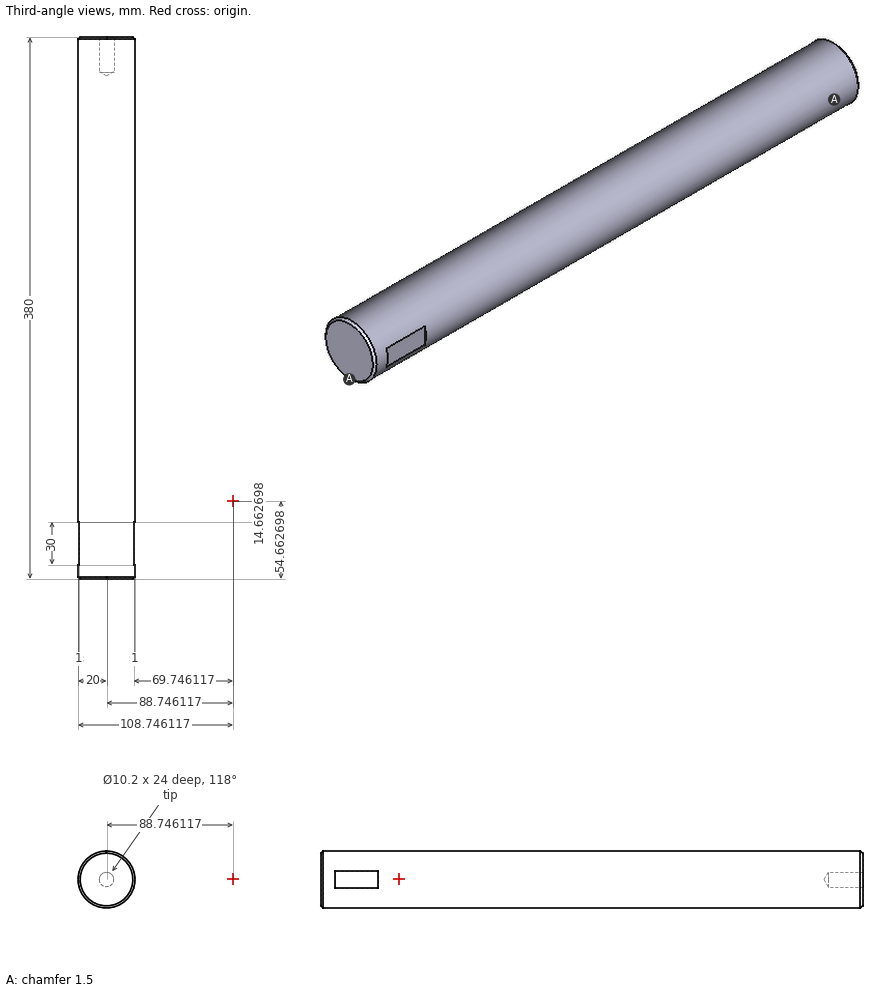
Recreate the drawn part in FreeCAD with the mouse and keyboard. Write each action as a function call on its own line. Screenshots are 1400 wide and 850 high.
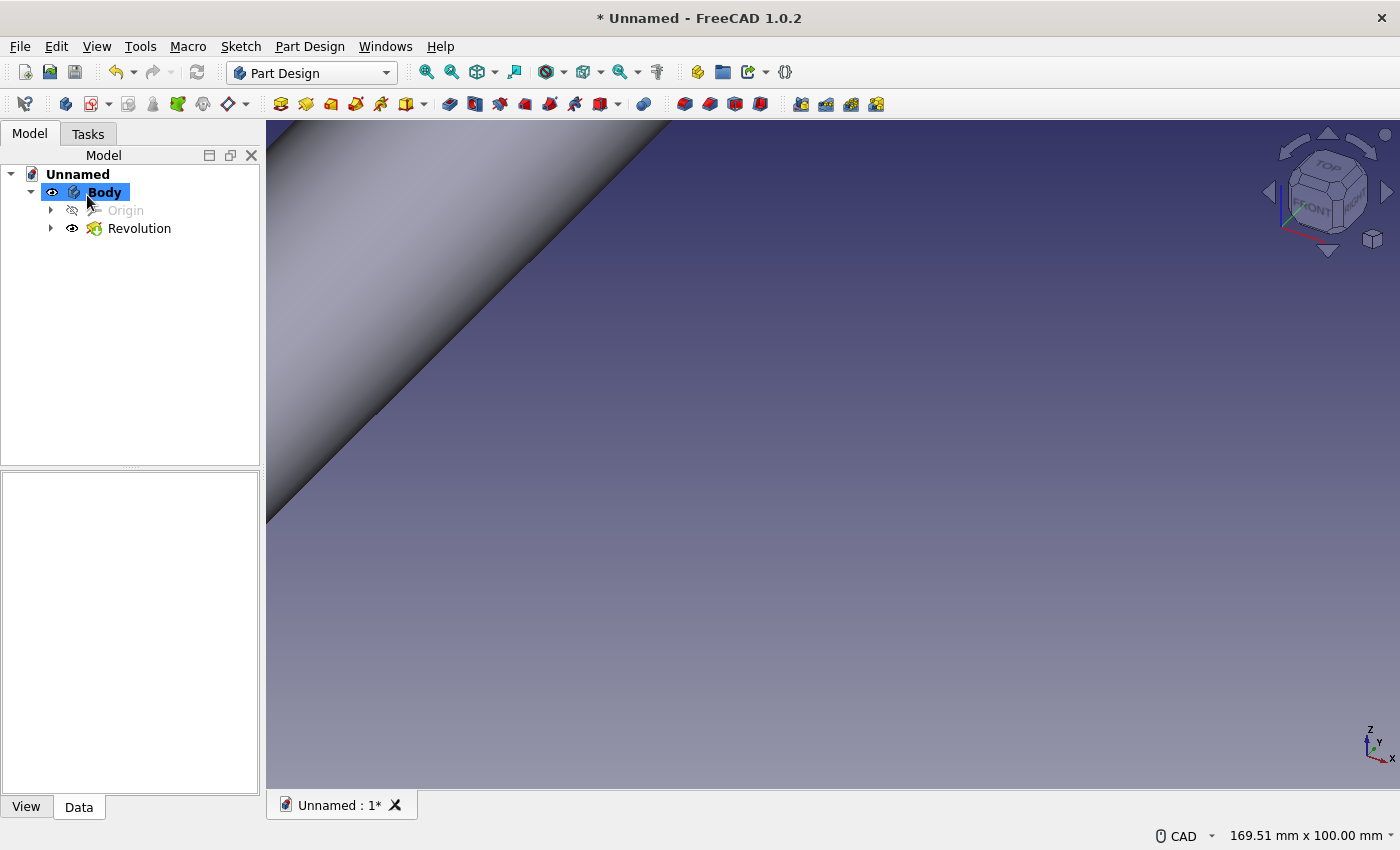
click(427, 72)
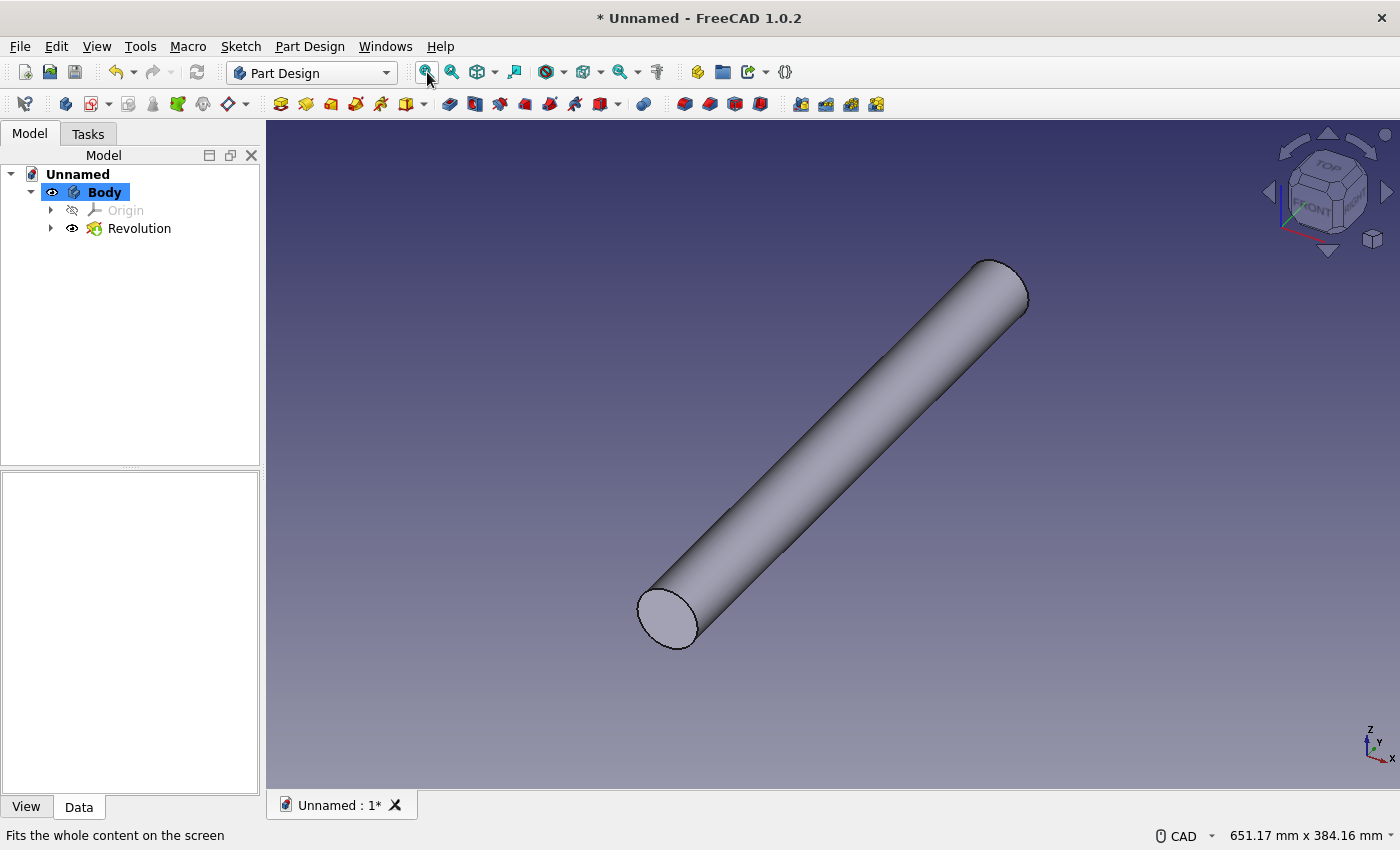
click(90, 104)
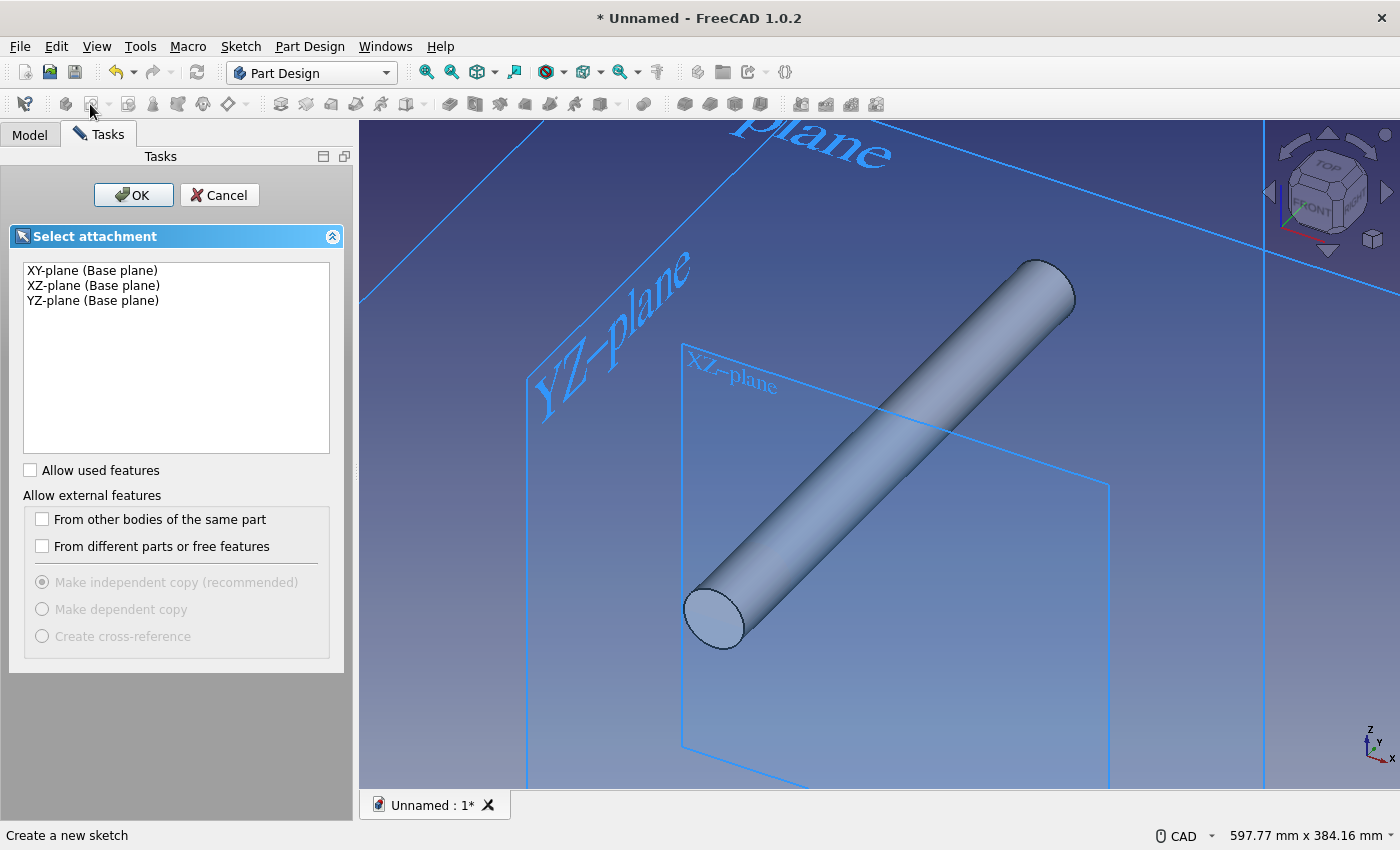
click(84, 270)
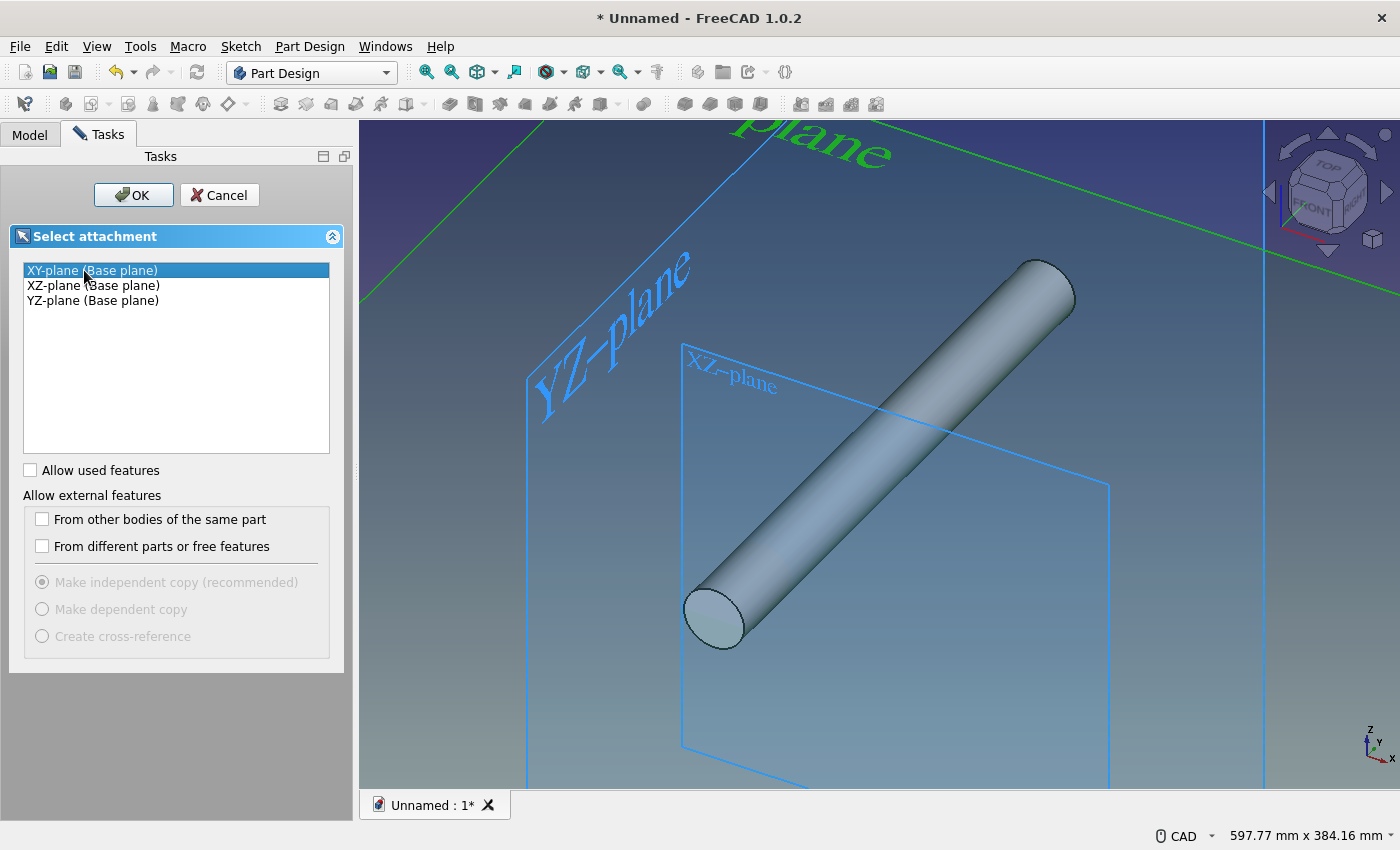
click(134, 195)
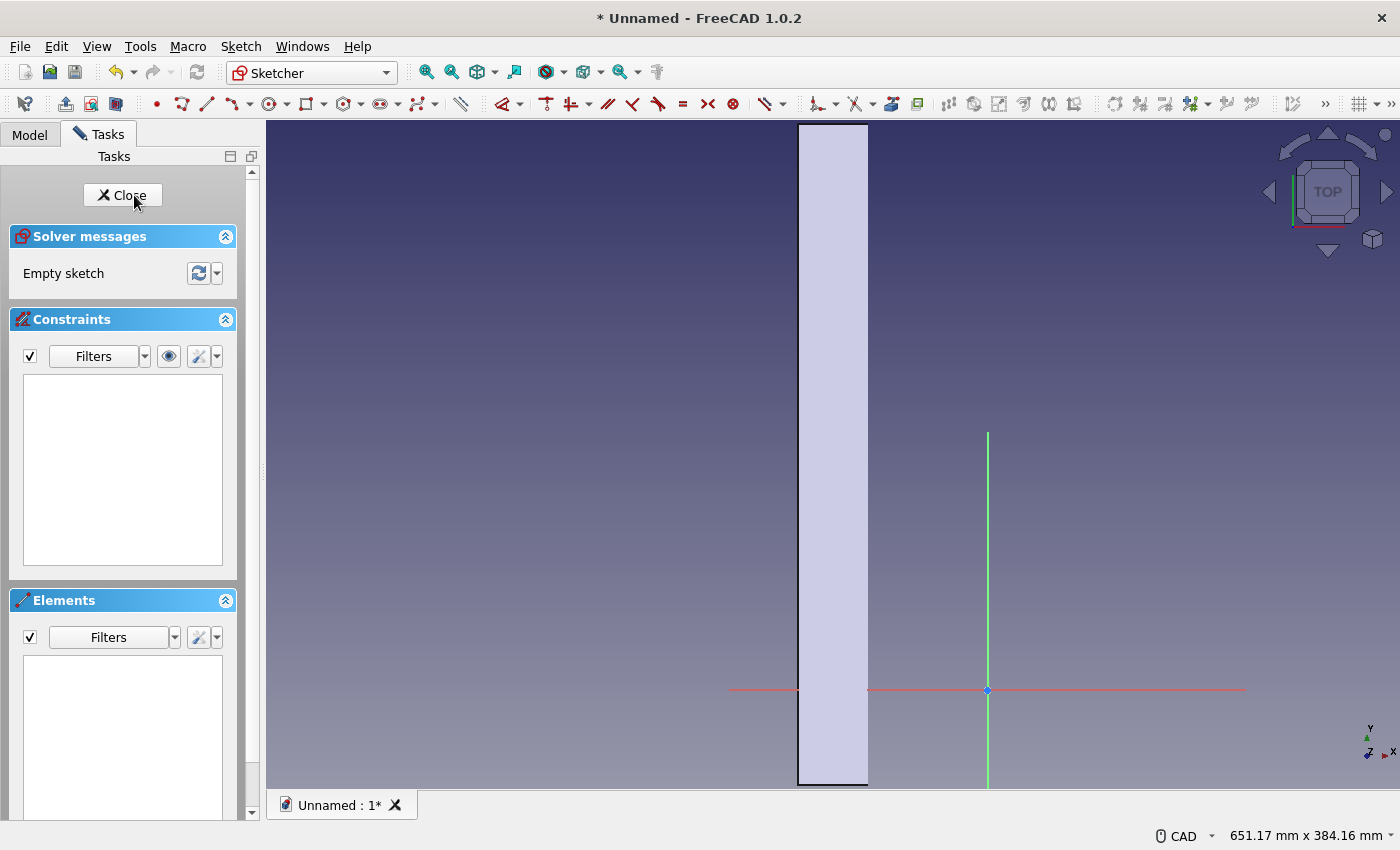
click(116, 104)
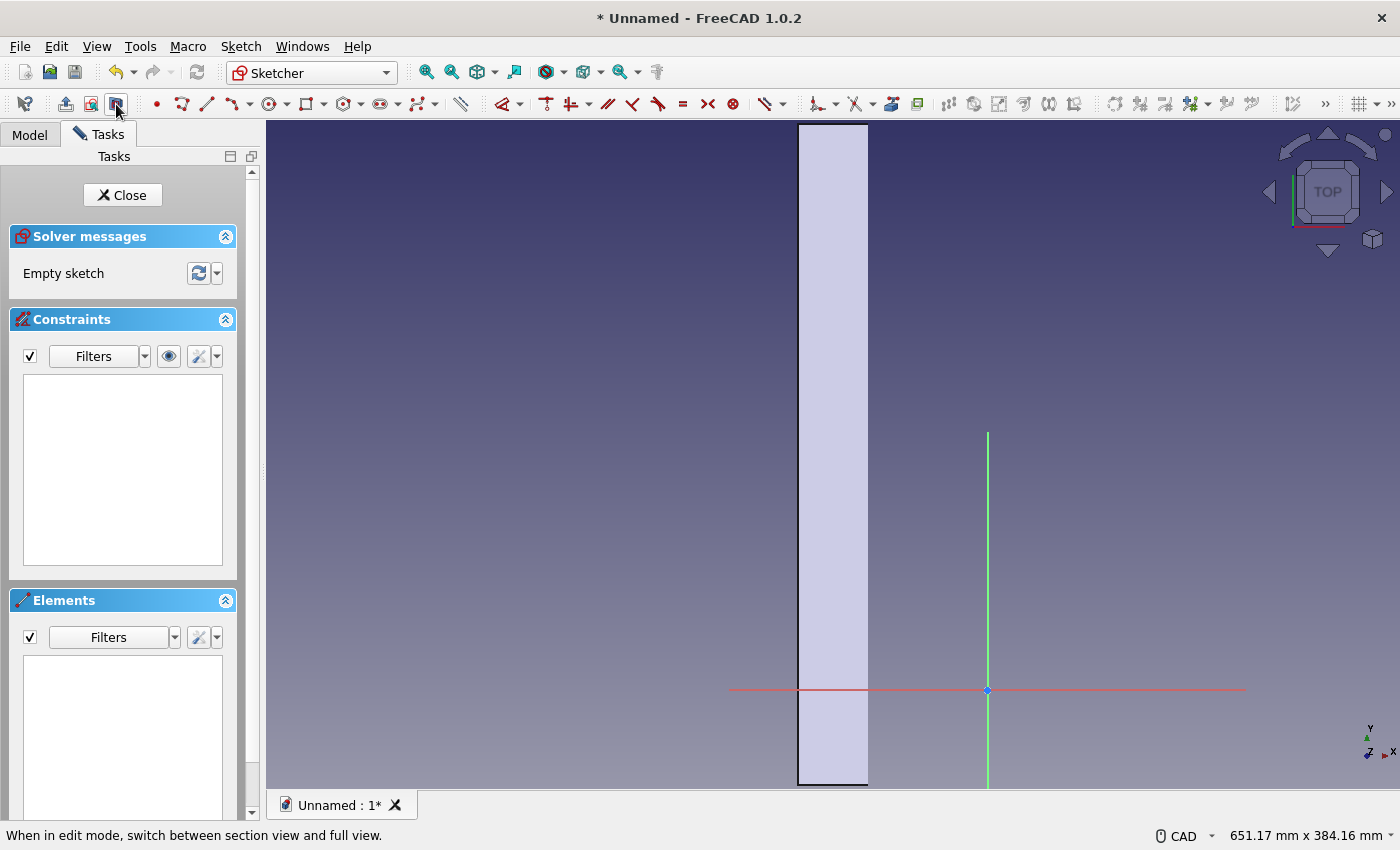
scroll(764, 454, down, 5)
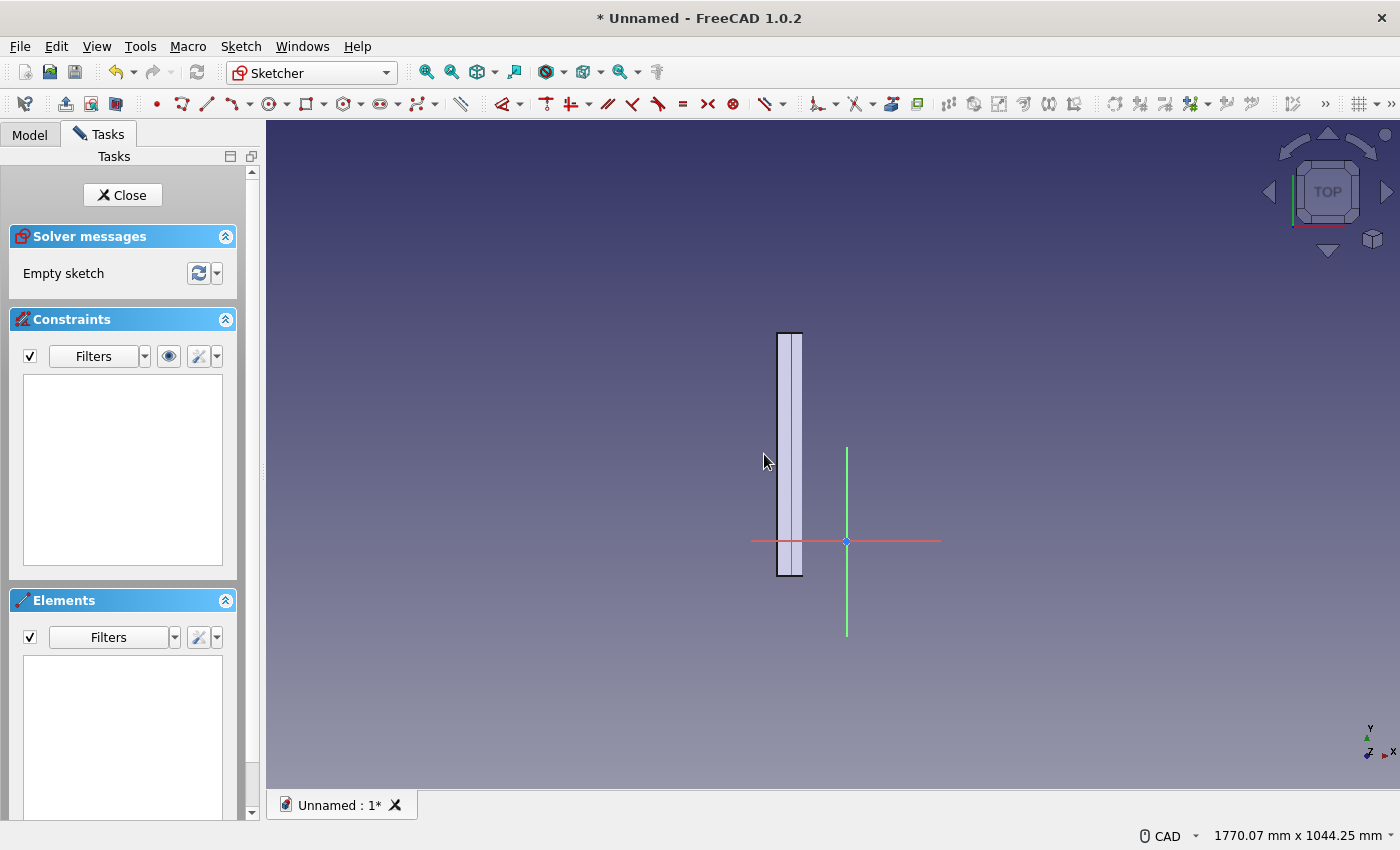
scroll(791, 566, up, 15)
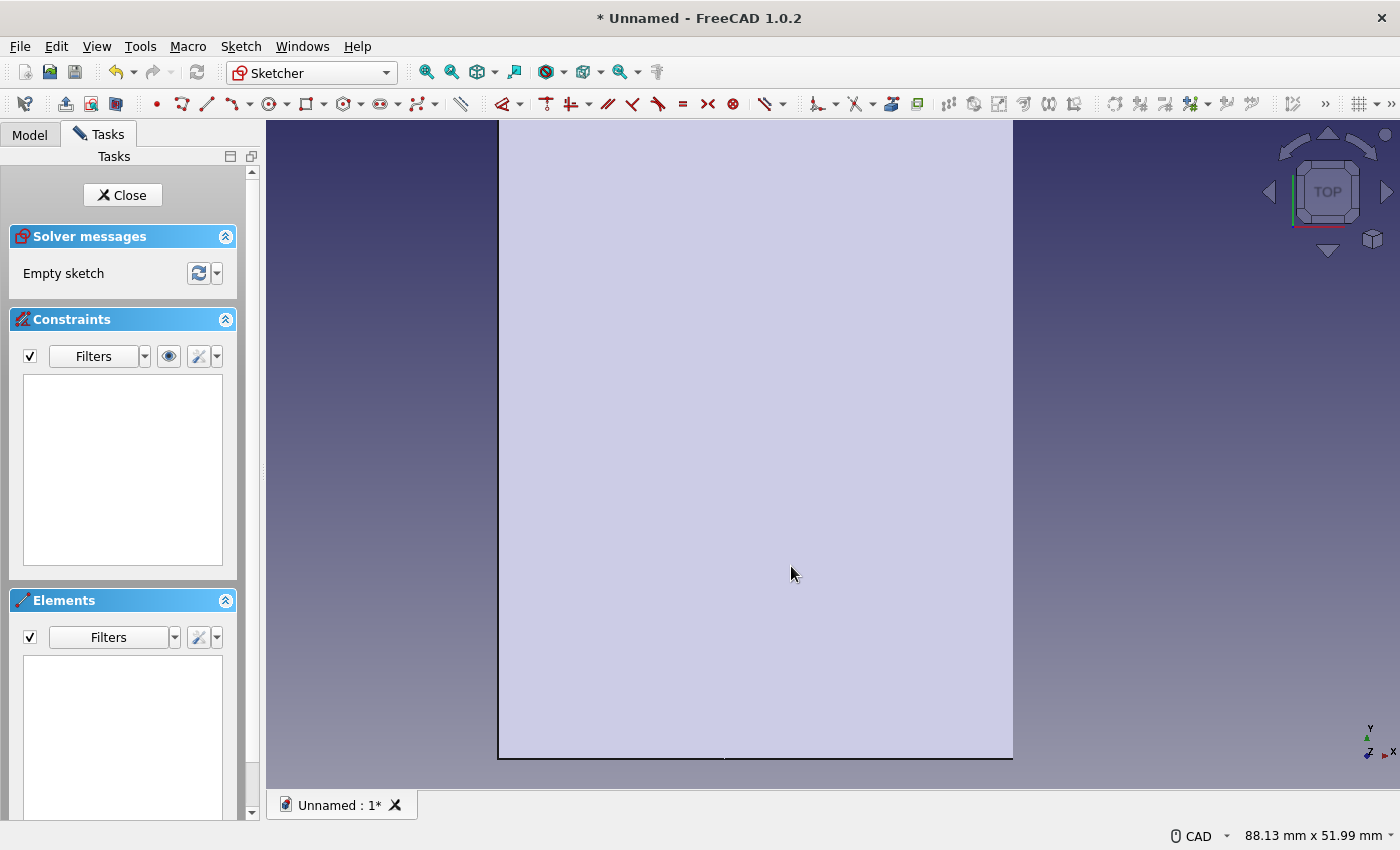
click(306, 104)